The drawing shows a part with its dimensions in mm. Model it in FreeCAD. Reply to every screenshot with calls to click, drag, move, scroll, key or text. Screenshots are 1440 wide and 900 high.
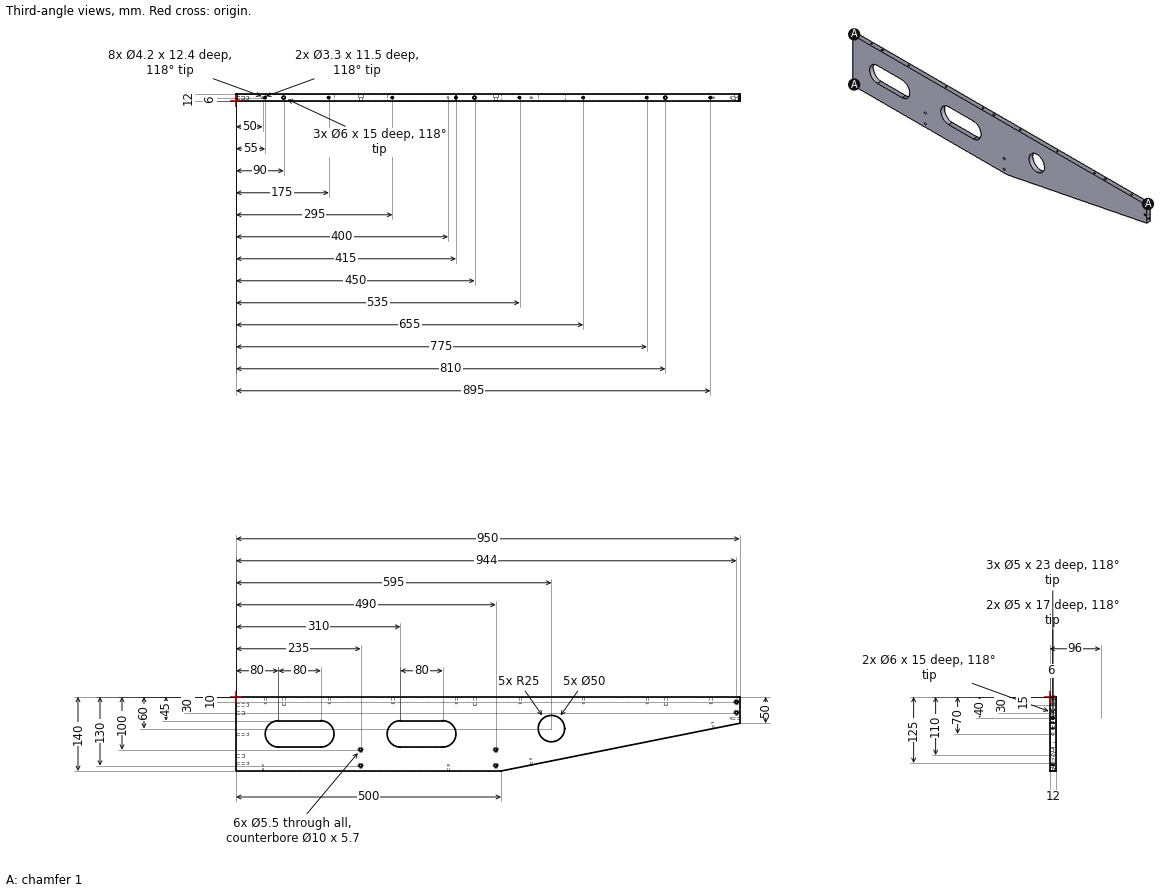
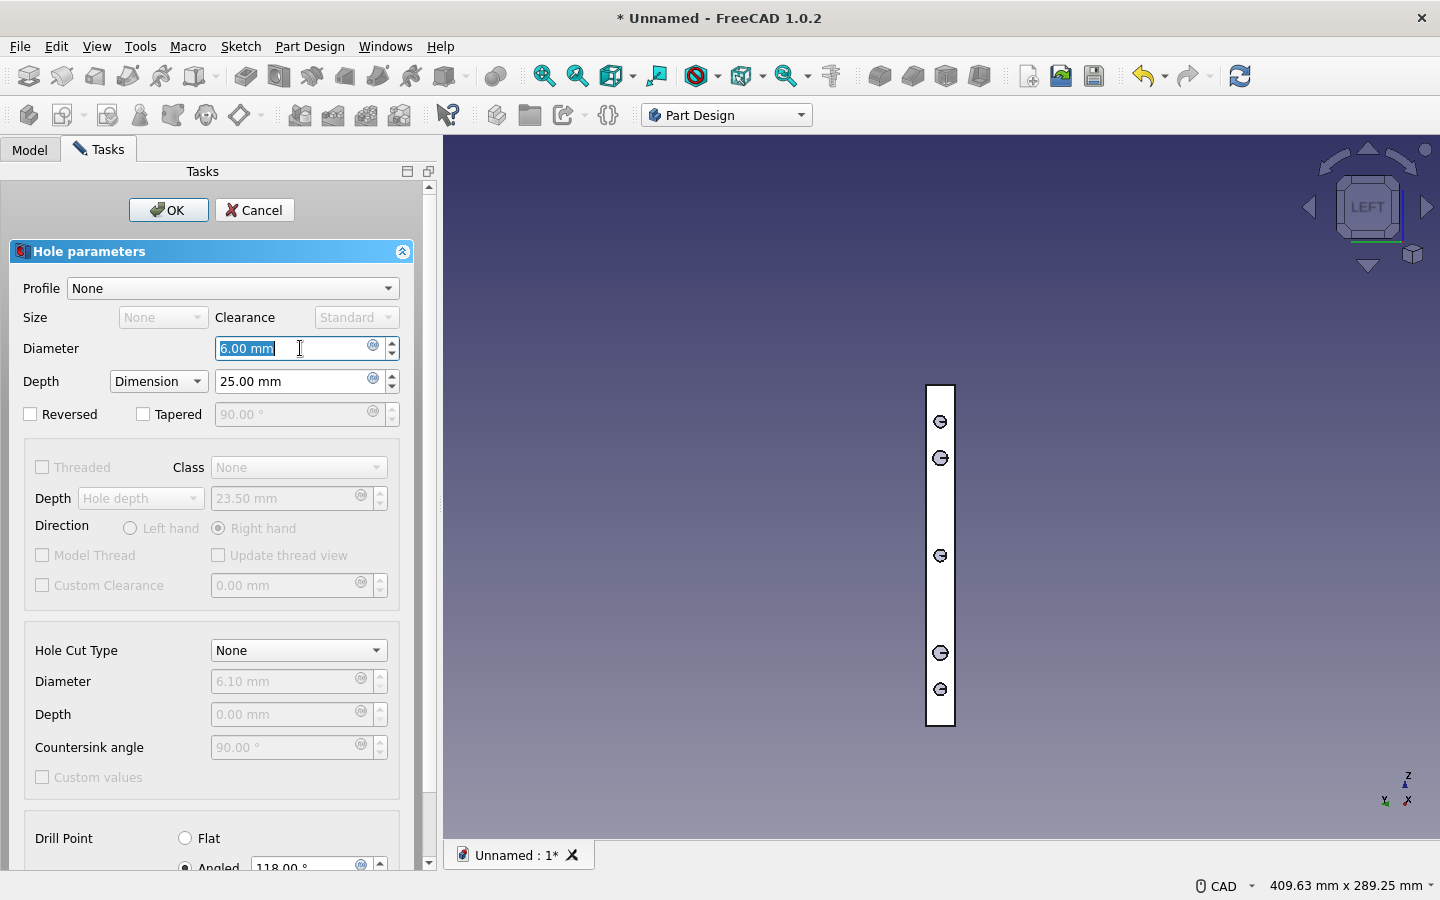
text(6)
key(Tab)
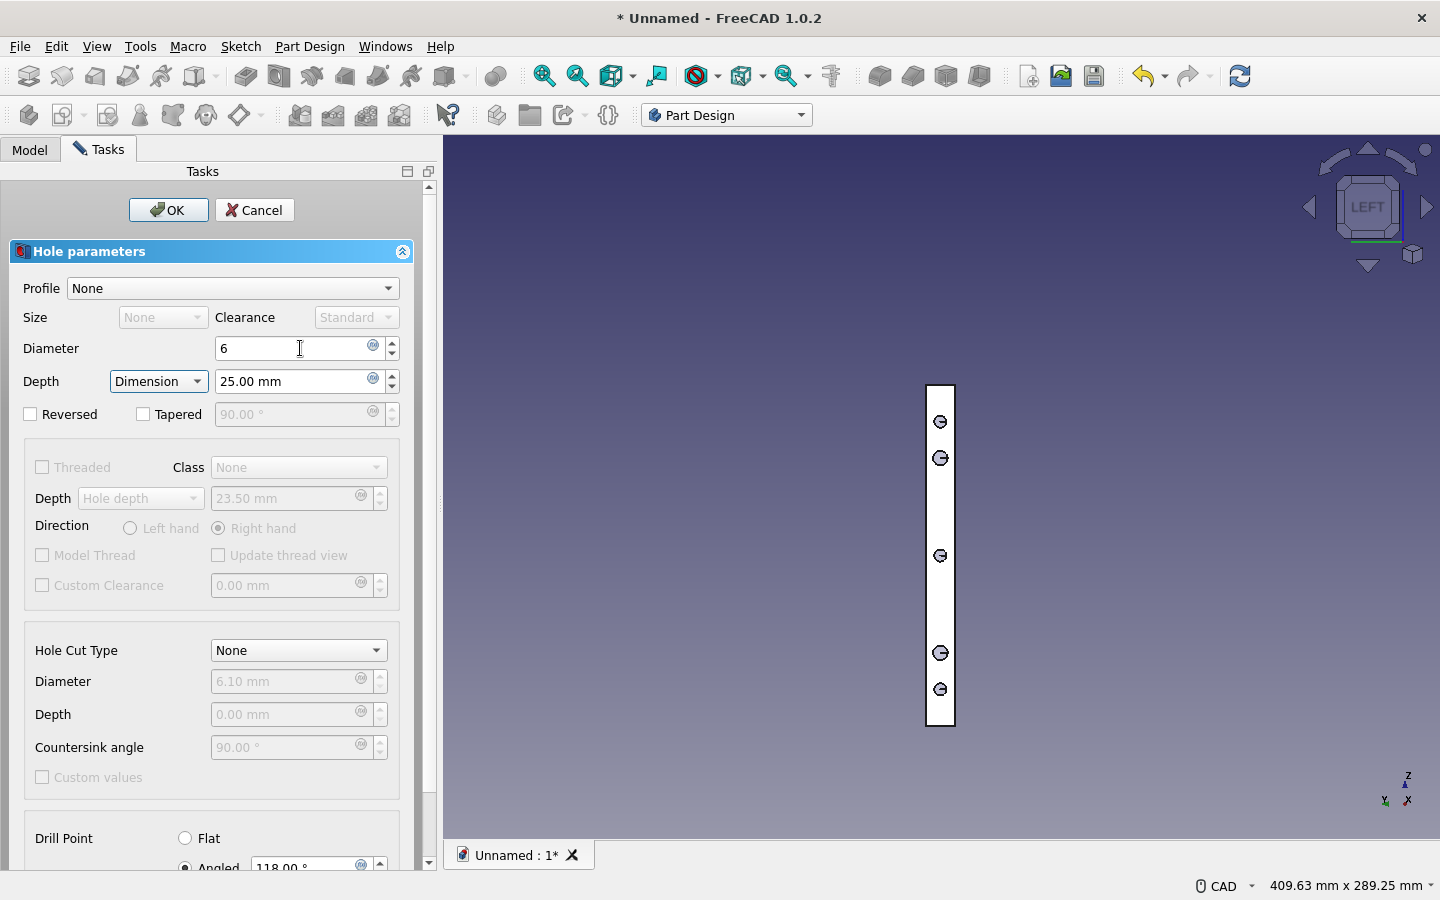
triple_click(300, 382)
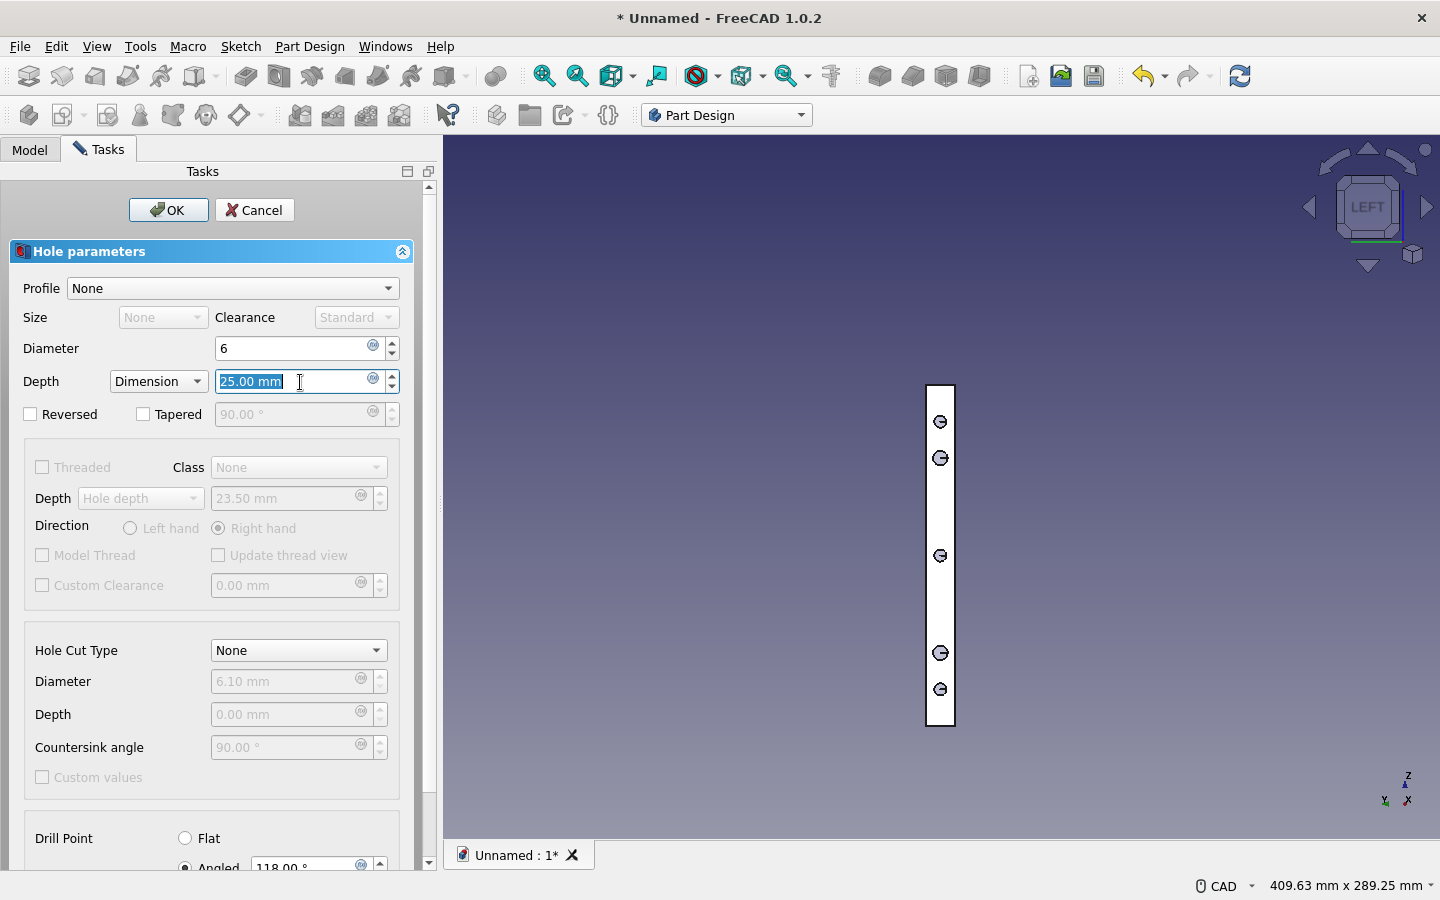
text(15)
key(Tab)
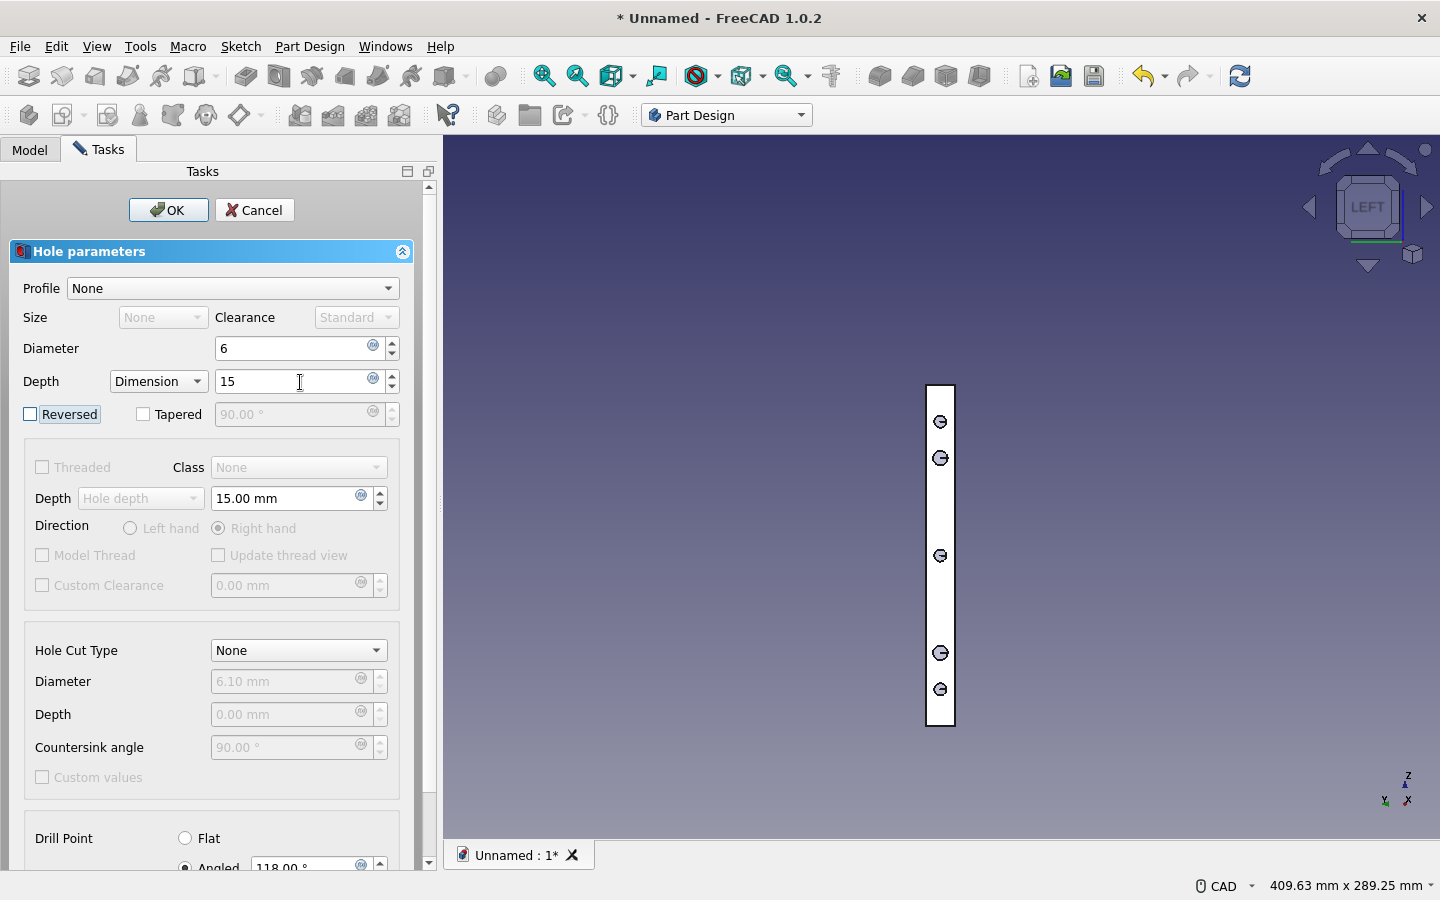
click(169, 210)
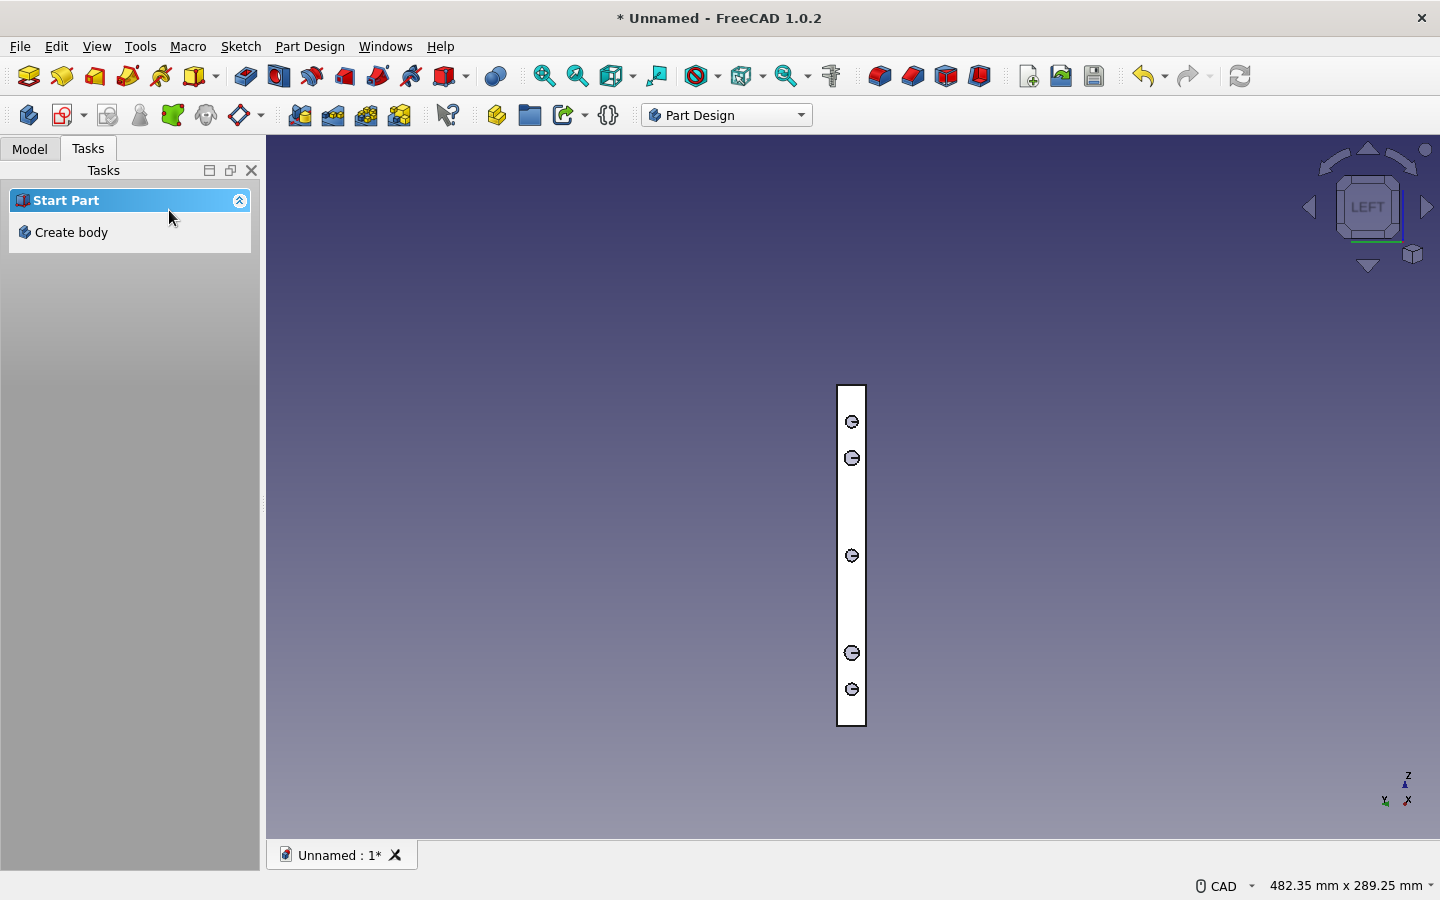
key(0)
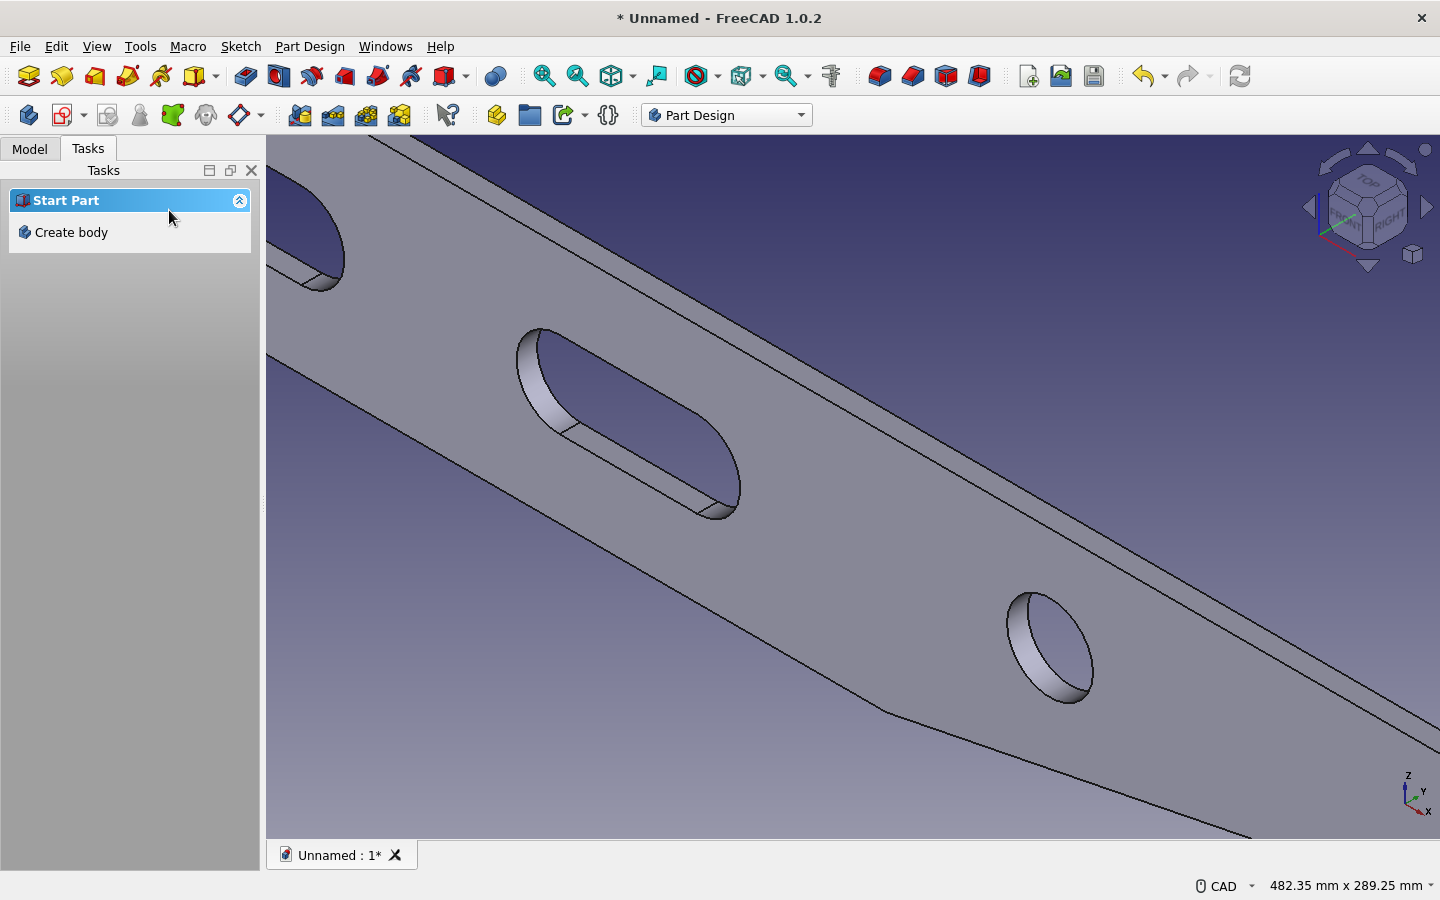
click(545, 76)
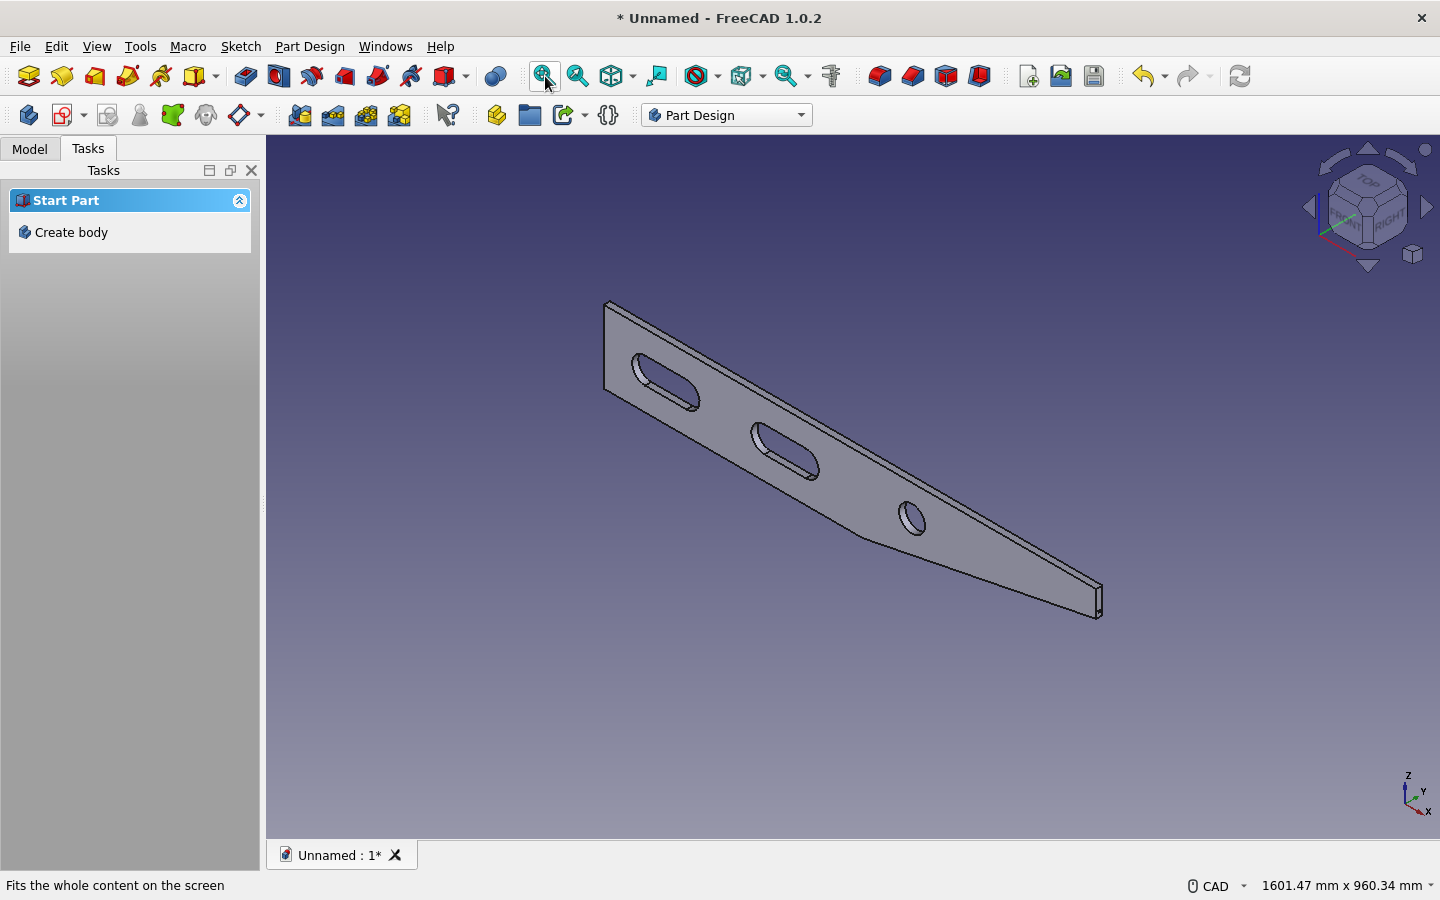
scroll(1064, 566, up, 6)